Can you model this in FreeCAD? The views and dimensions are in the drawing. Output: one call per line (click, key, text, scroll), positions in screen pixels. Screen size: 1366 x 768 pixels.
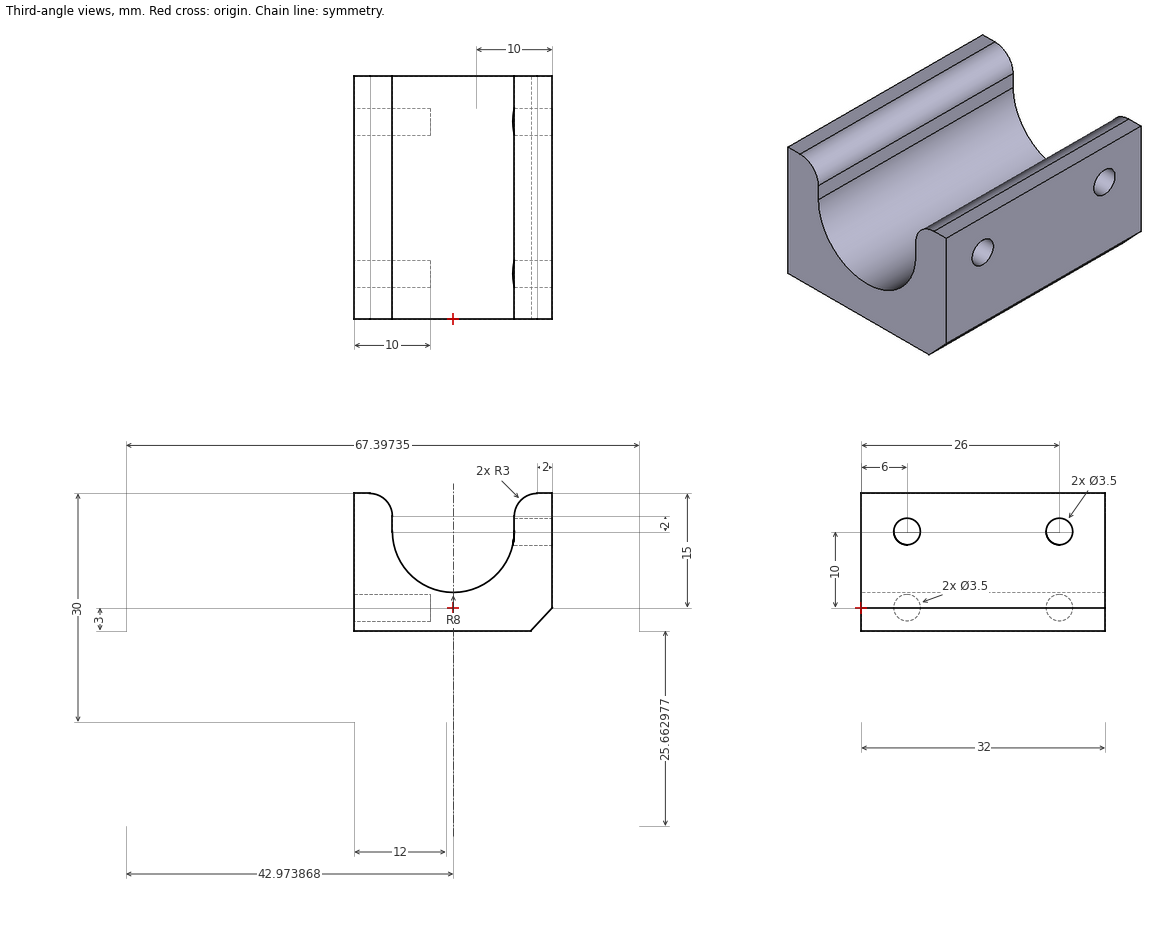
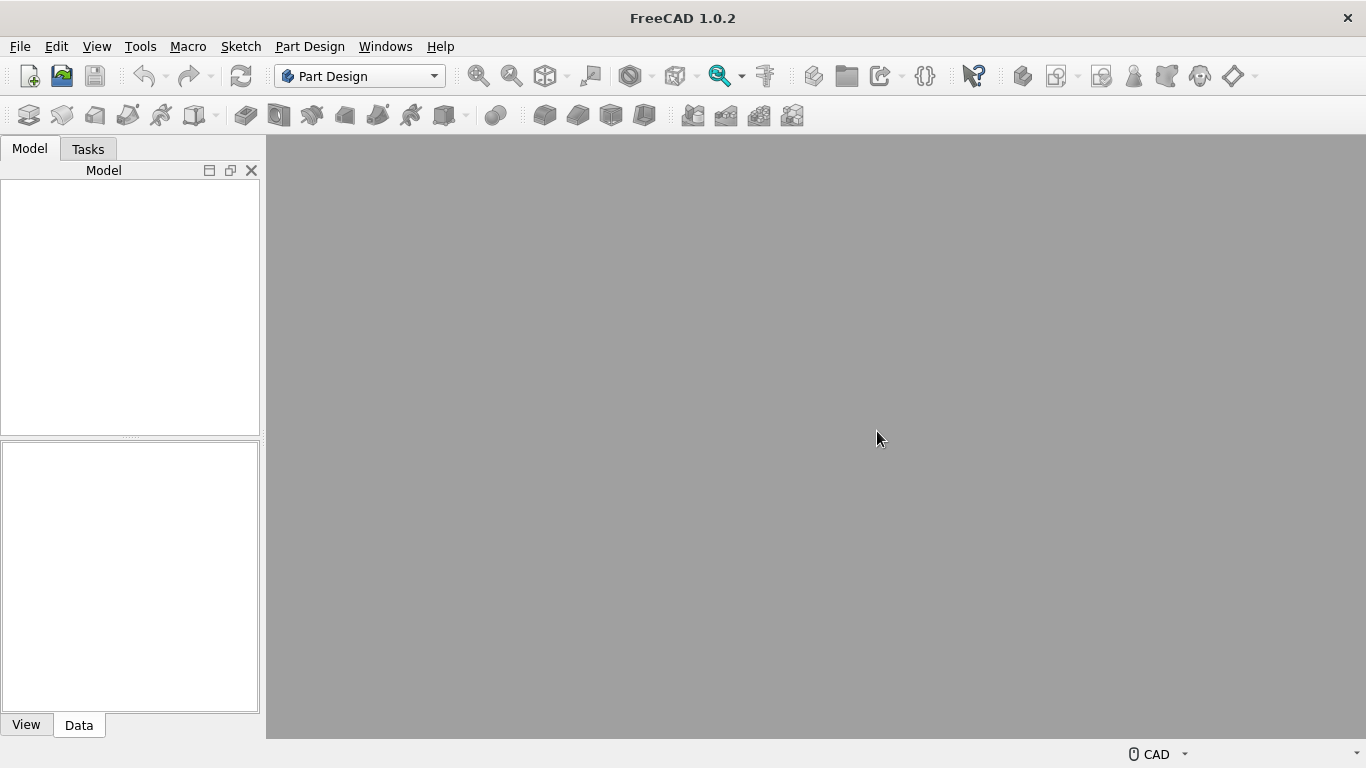
click(29, 76)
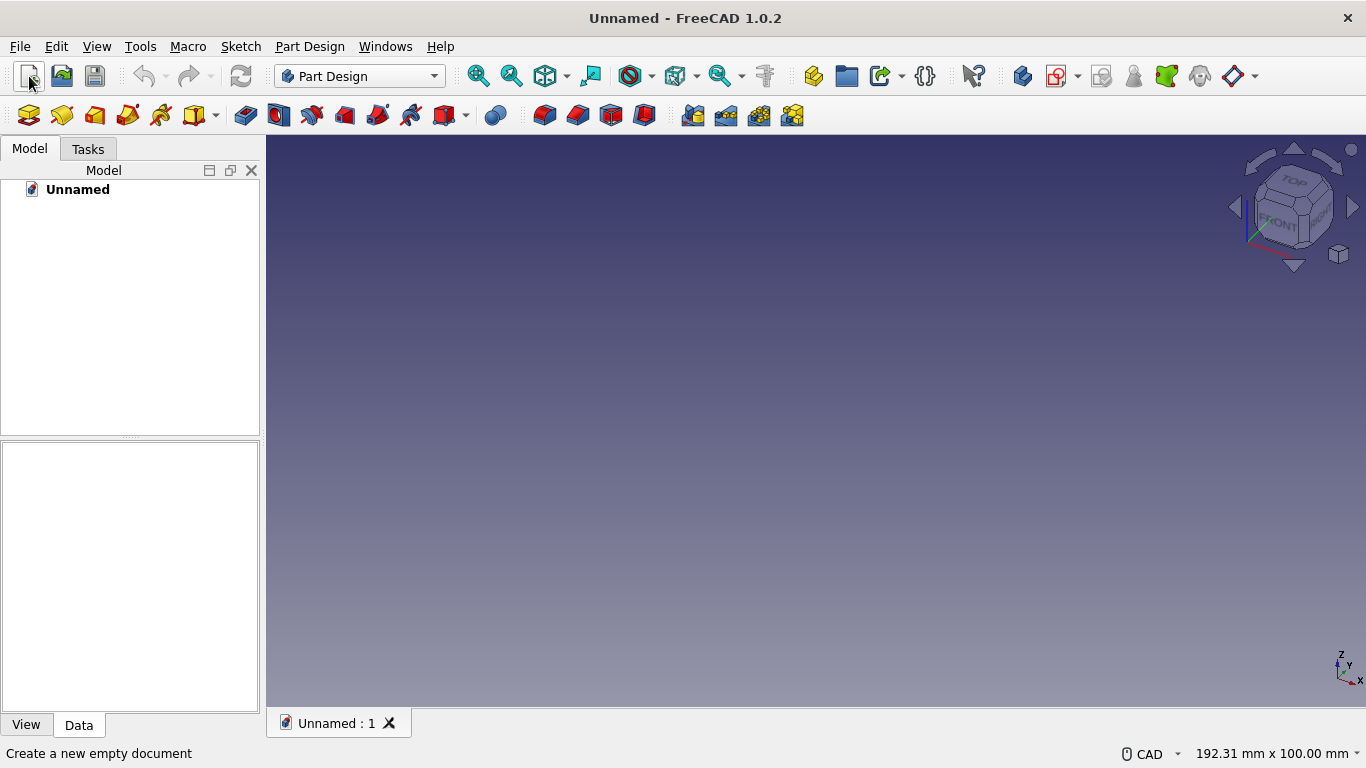
click(1056, 76)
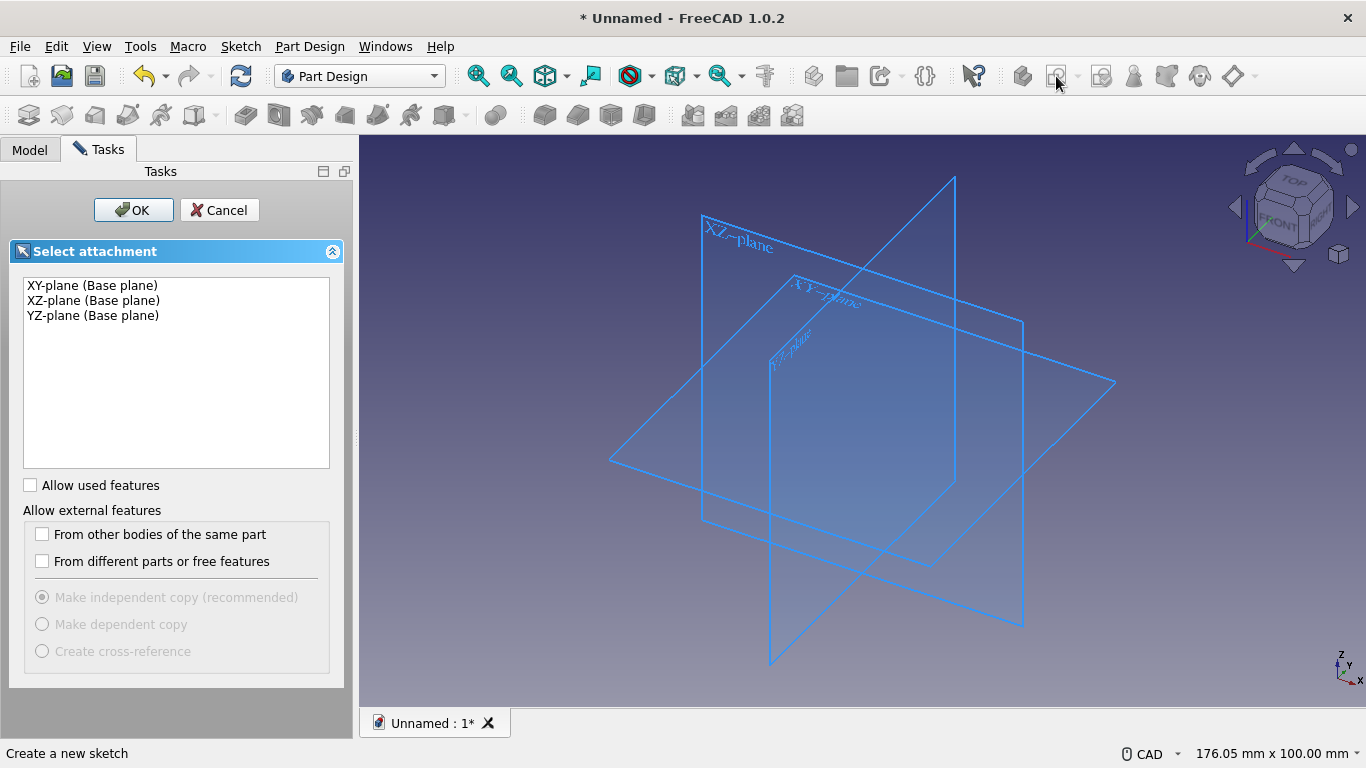
click(84, 300)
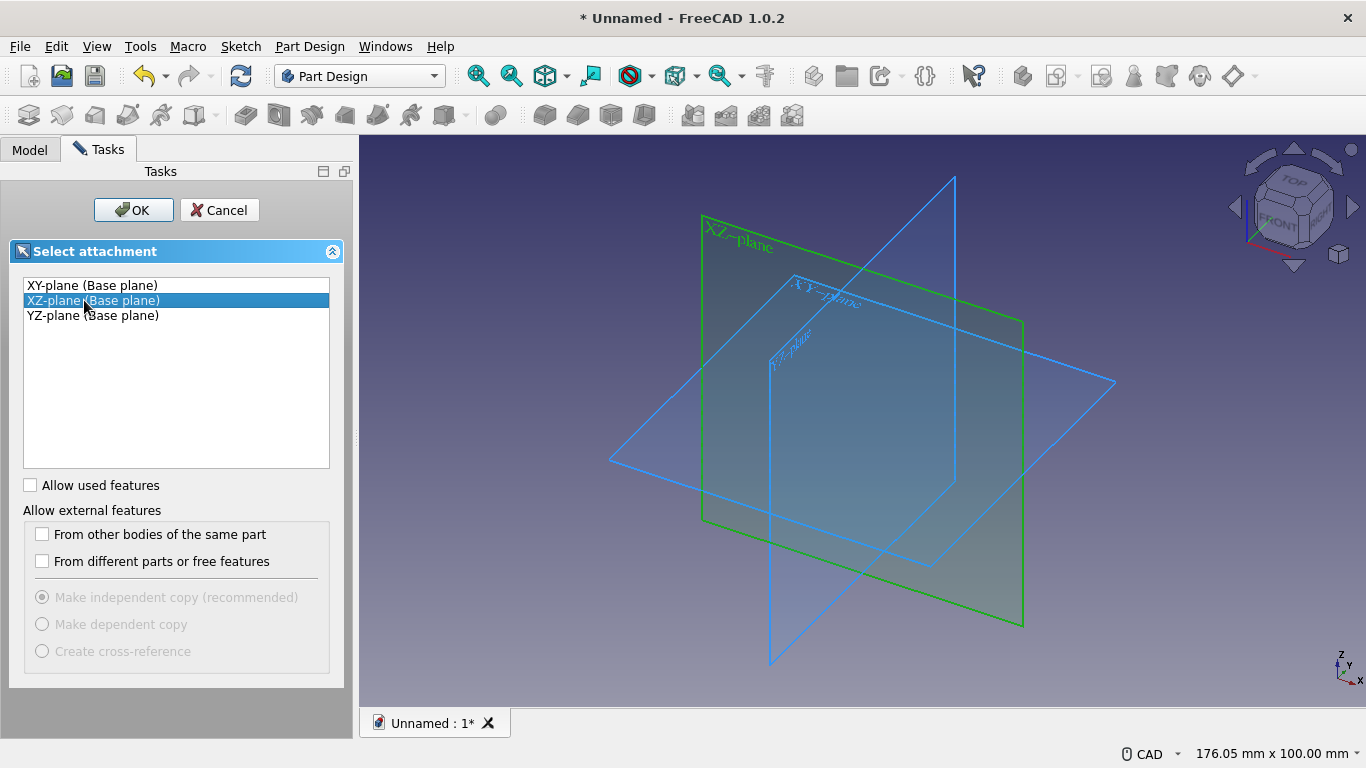
click(134, 210)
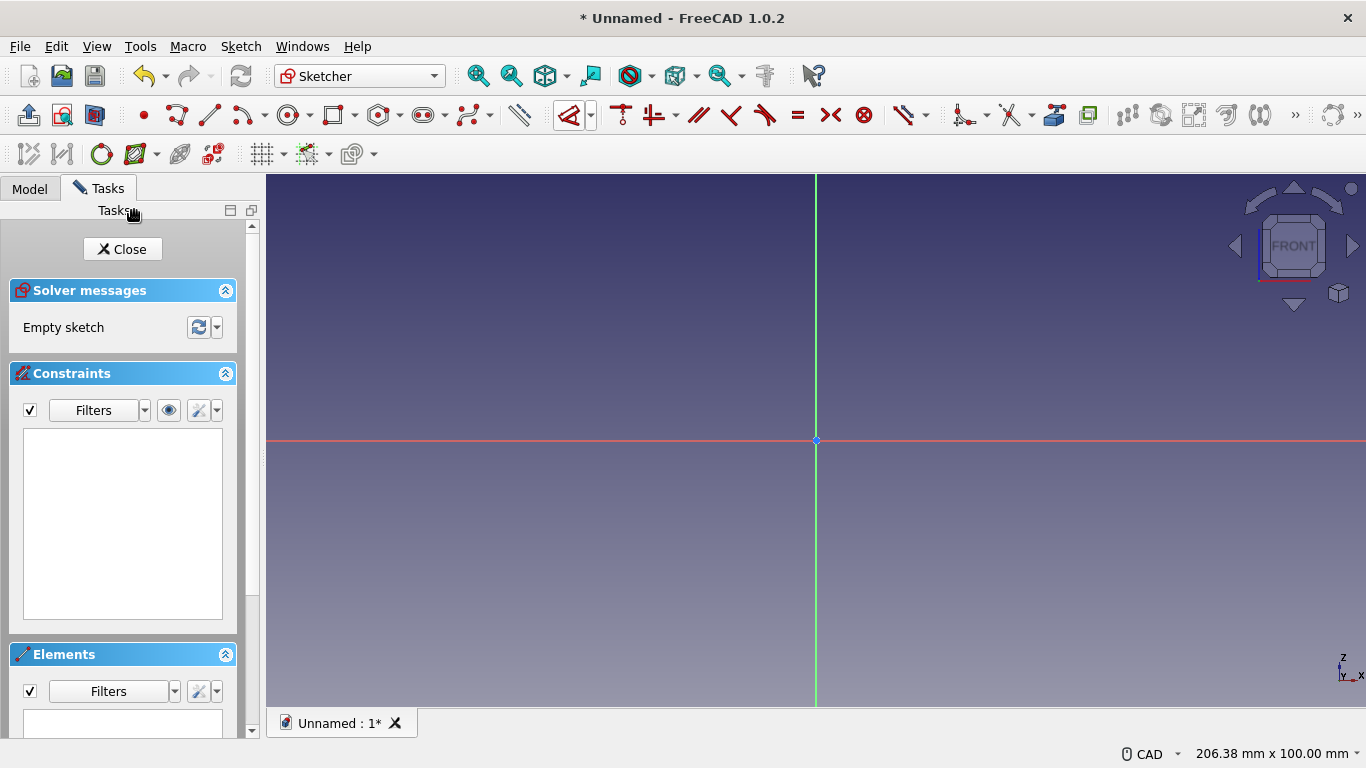
scroll(872, 440, up, 4)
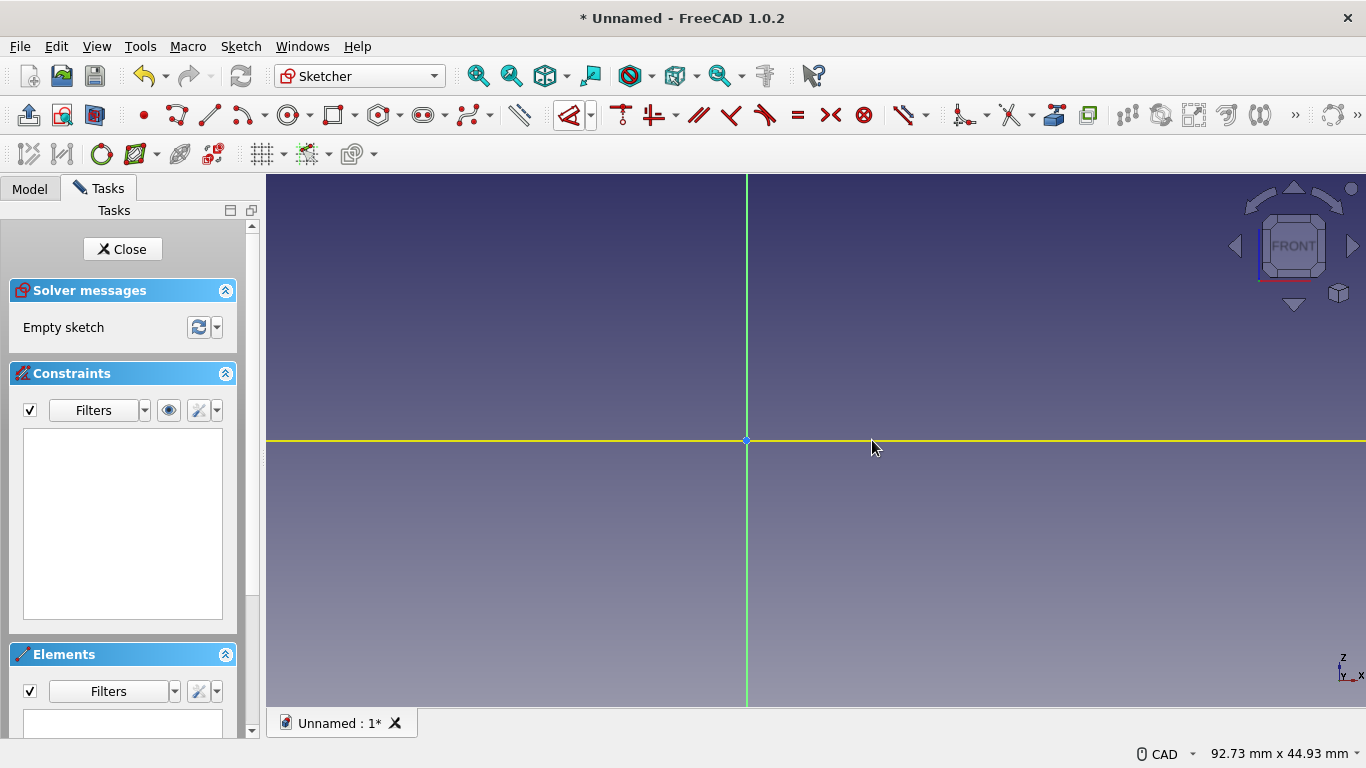
click(210, 116)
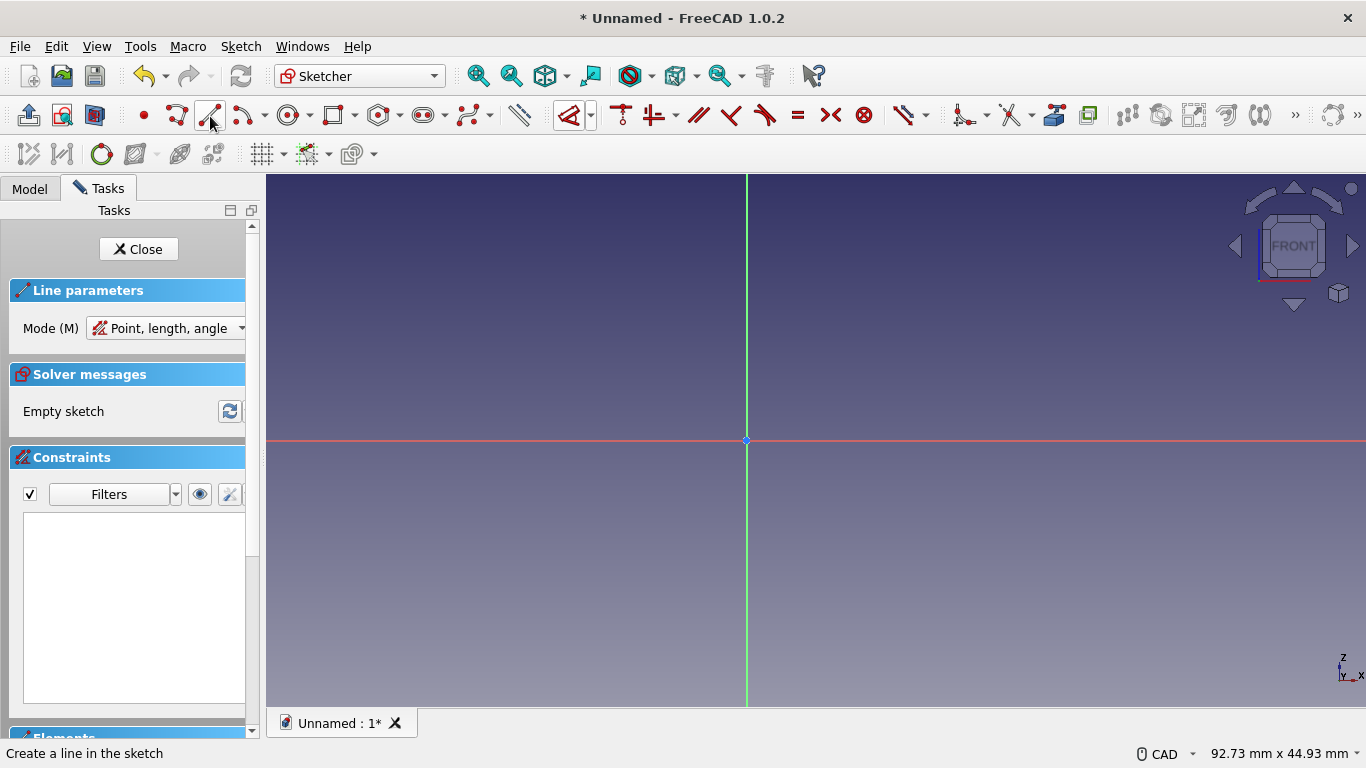
click(652, 298)
click(652, 322)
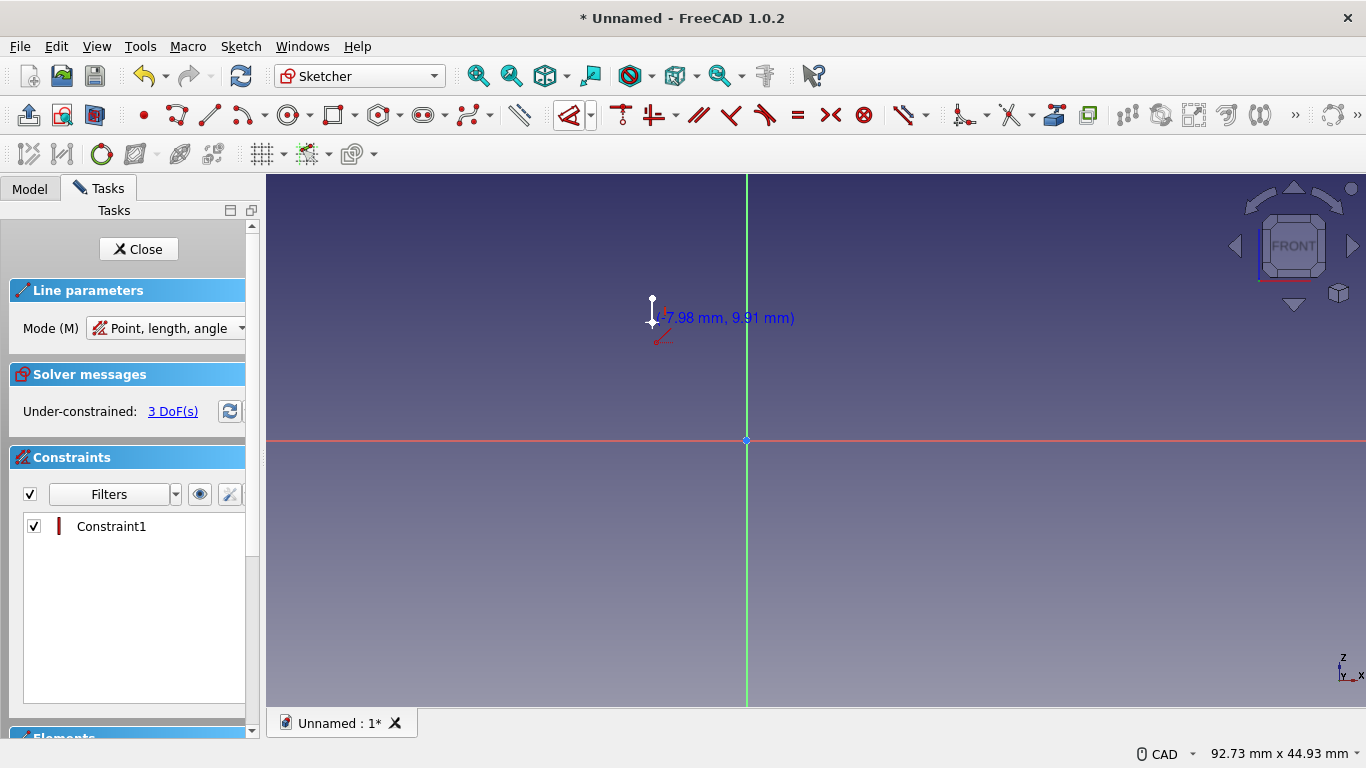
click(842, 322)
click(842, 298)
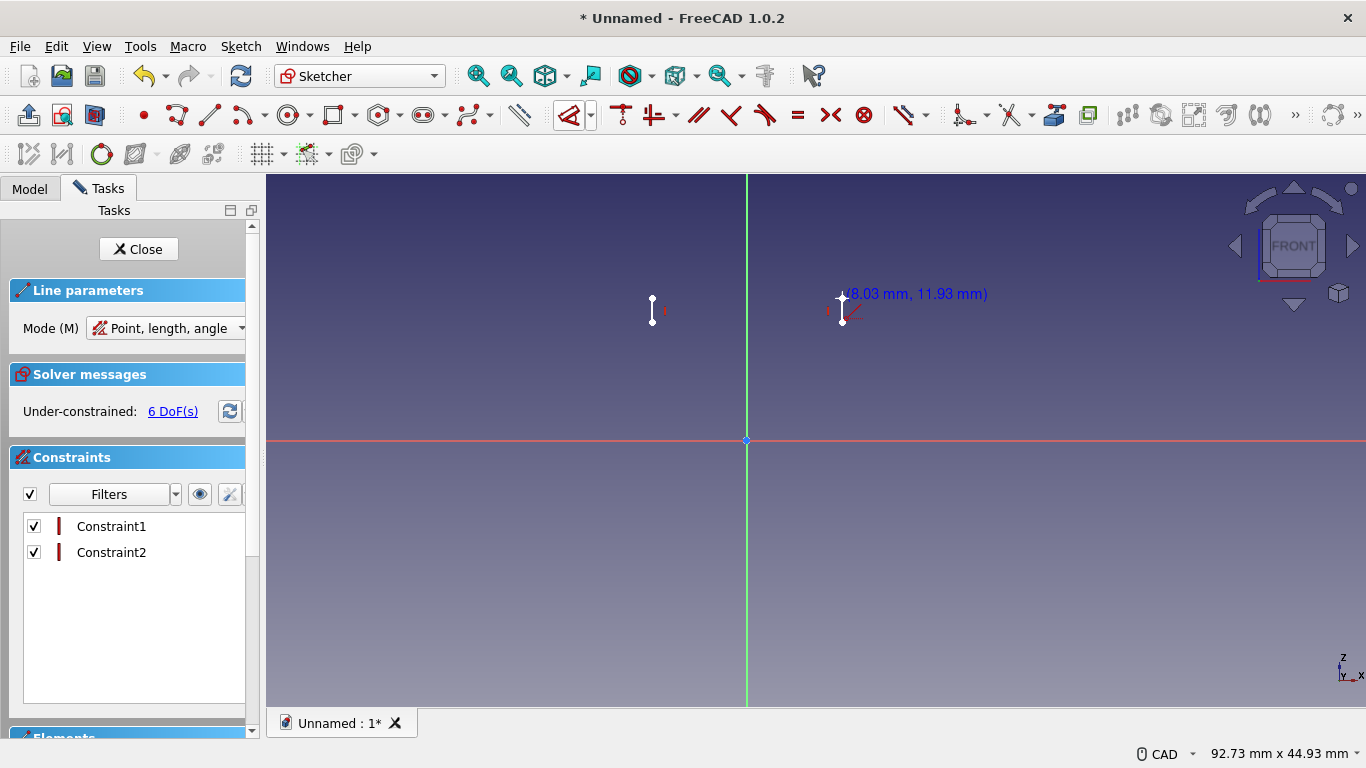
click(177, 116)